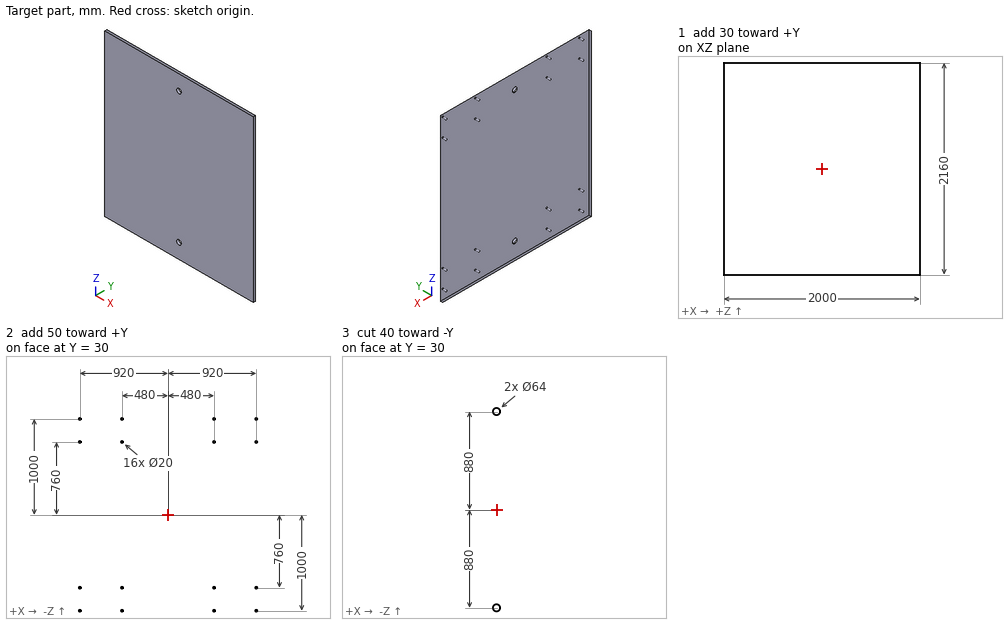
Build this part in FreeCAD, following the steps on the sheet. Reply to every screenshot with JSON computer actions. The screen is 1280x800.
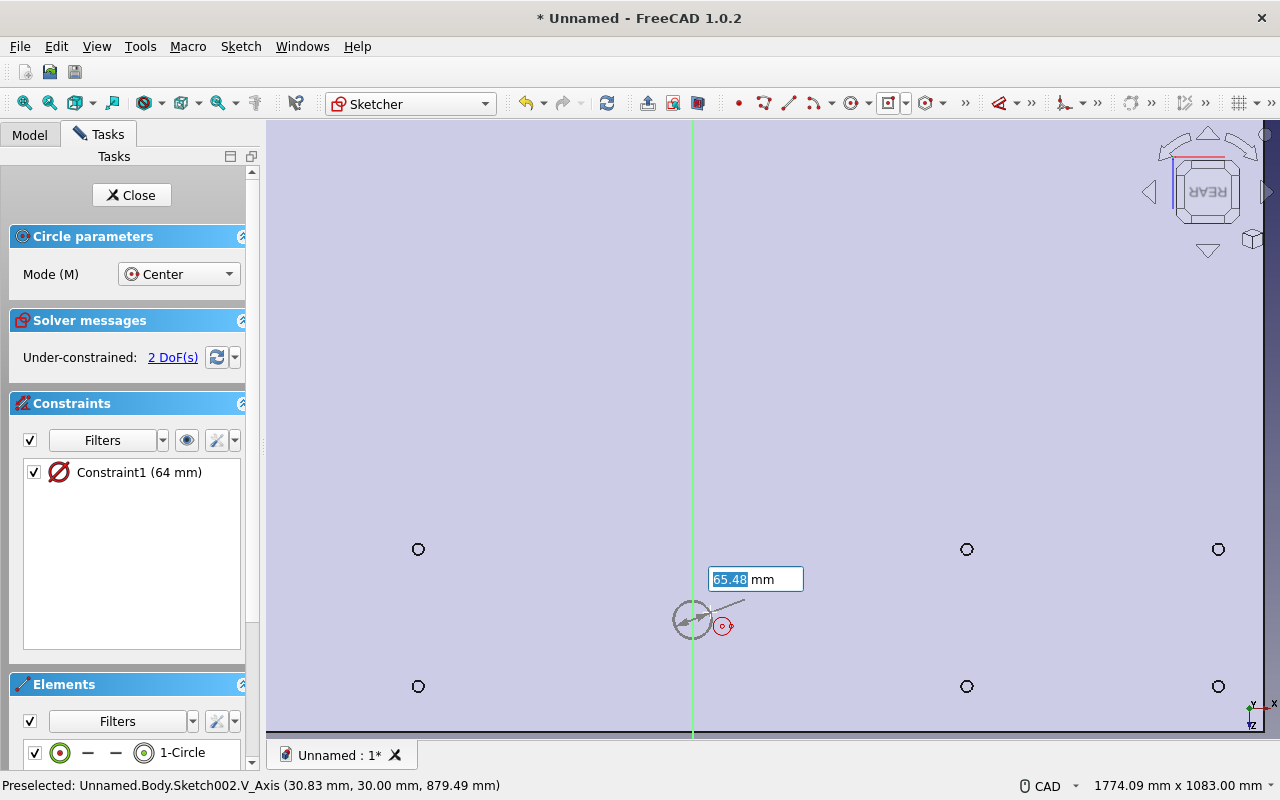
{"action": "type", "text": "64"}
{"action": "key", "text": "Return"}
{"action": "key", "text": "Escape"}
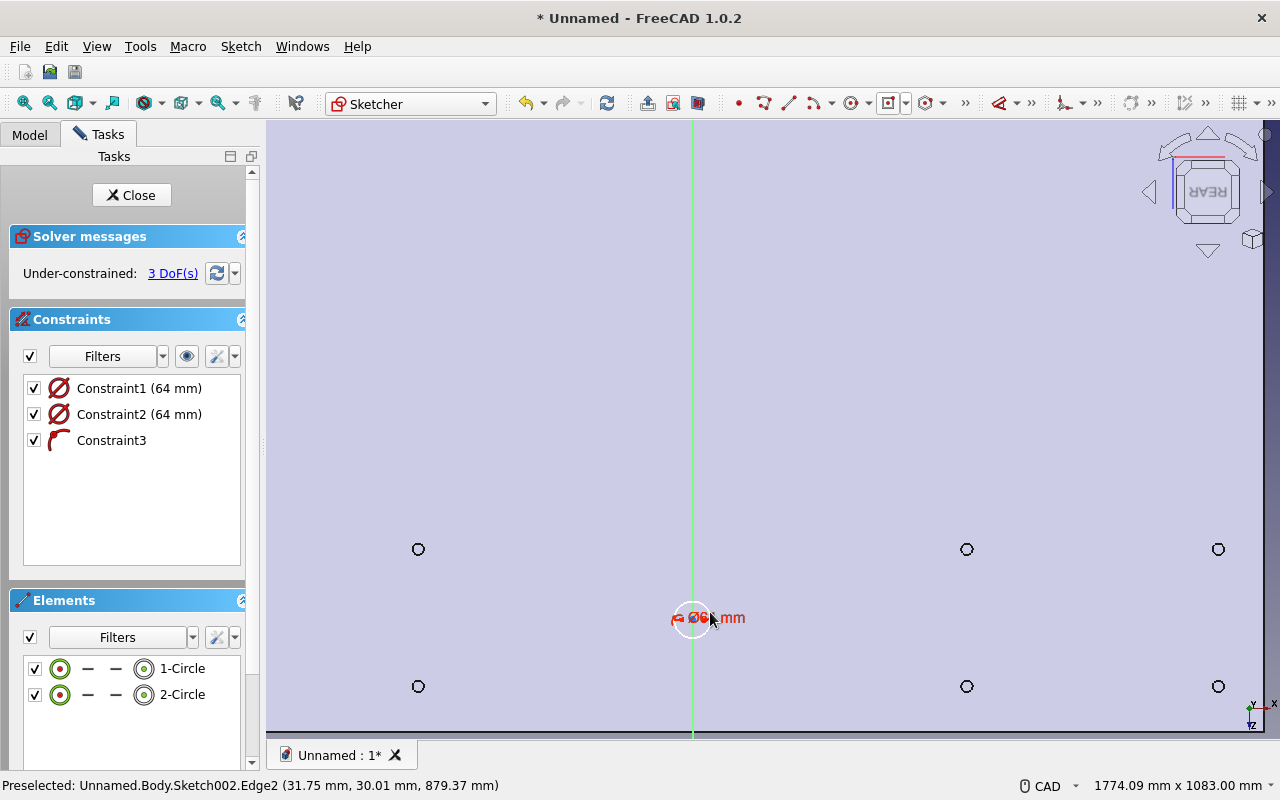
{"action": "scroll", "coordinate": [711, 613], "scroll_direction": "down", "scroll_amount": 5}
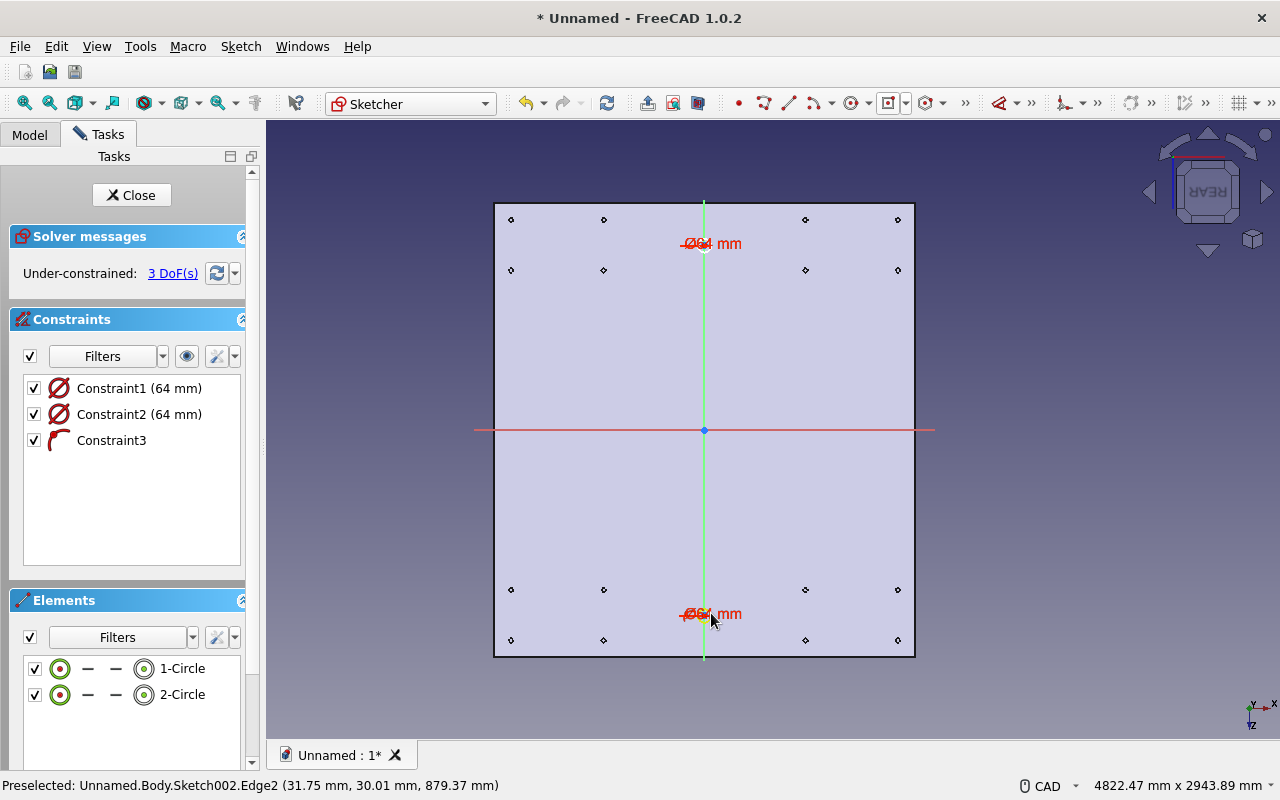
{"action": "left_click", "coordinate": [704, 246]}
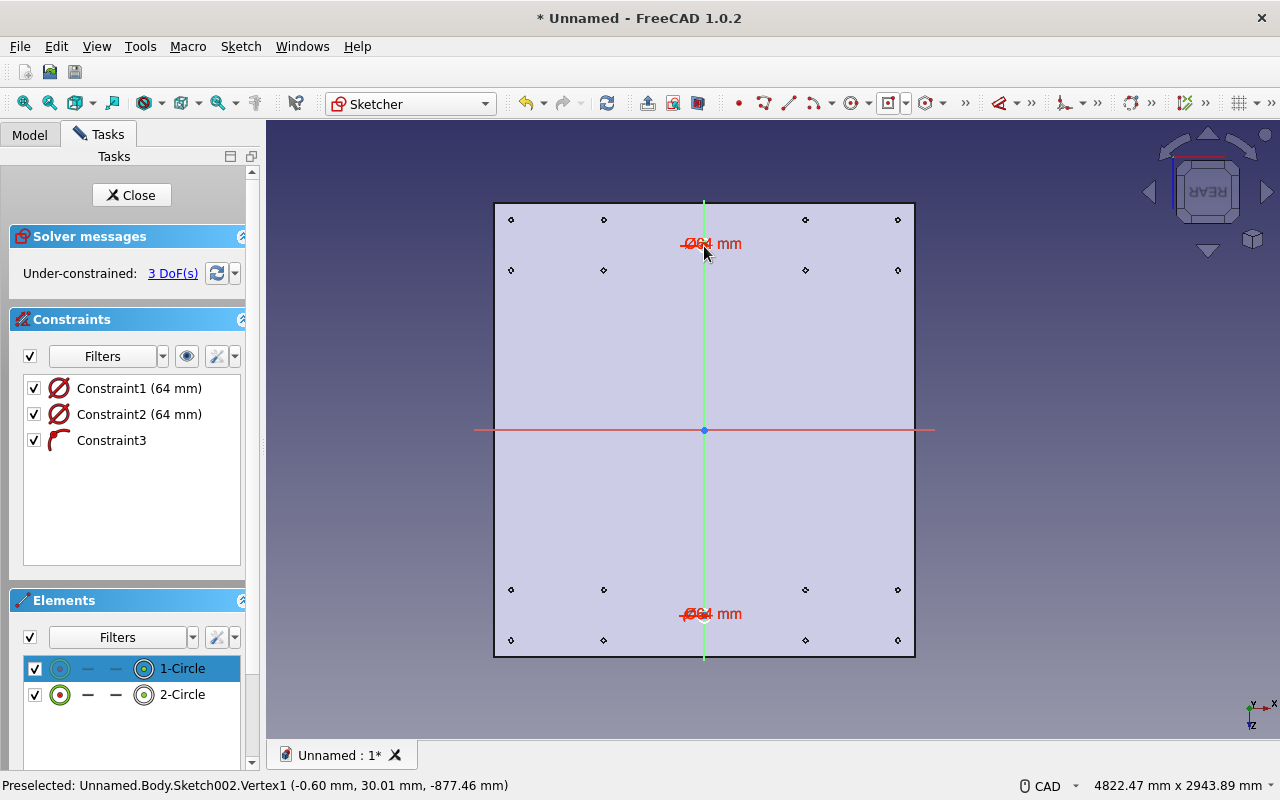
{"action": "left_click", "coordinate": [704, 550]}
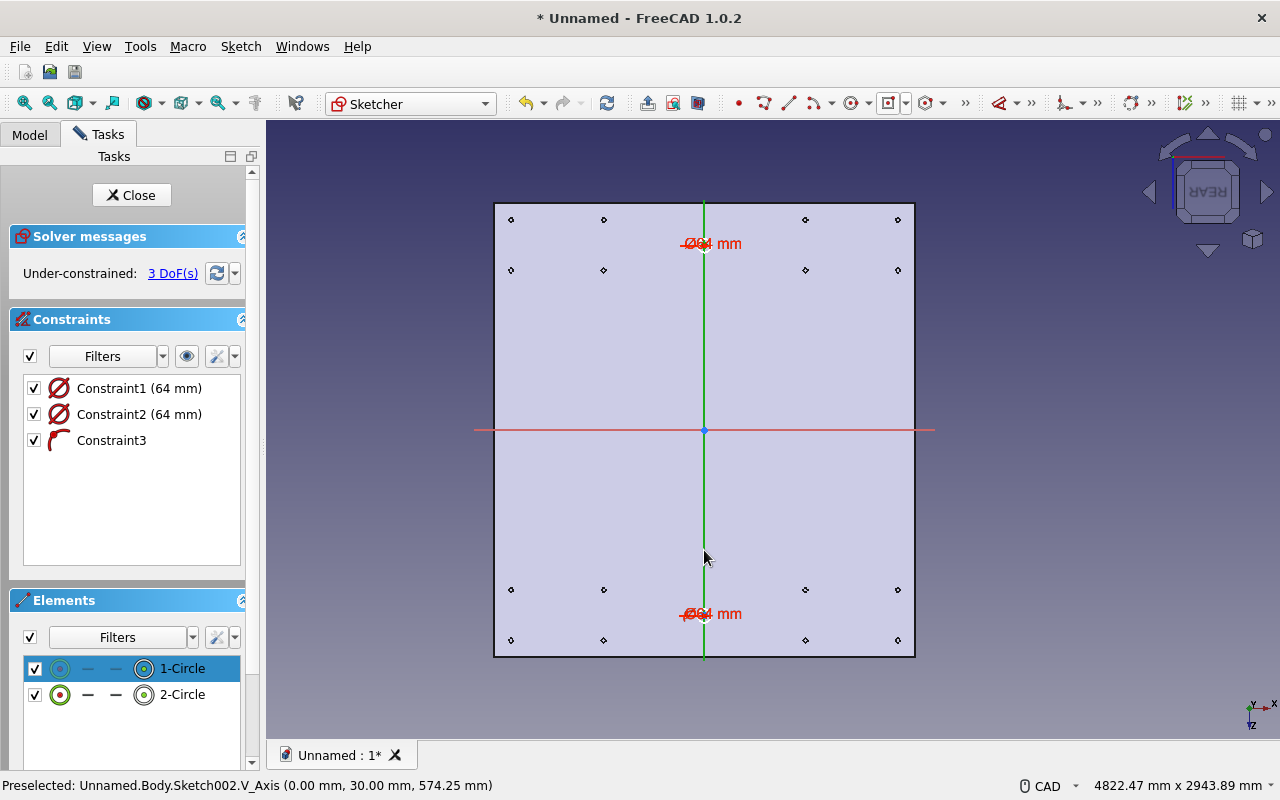
{"action": "key", "text": "c"}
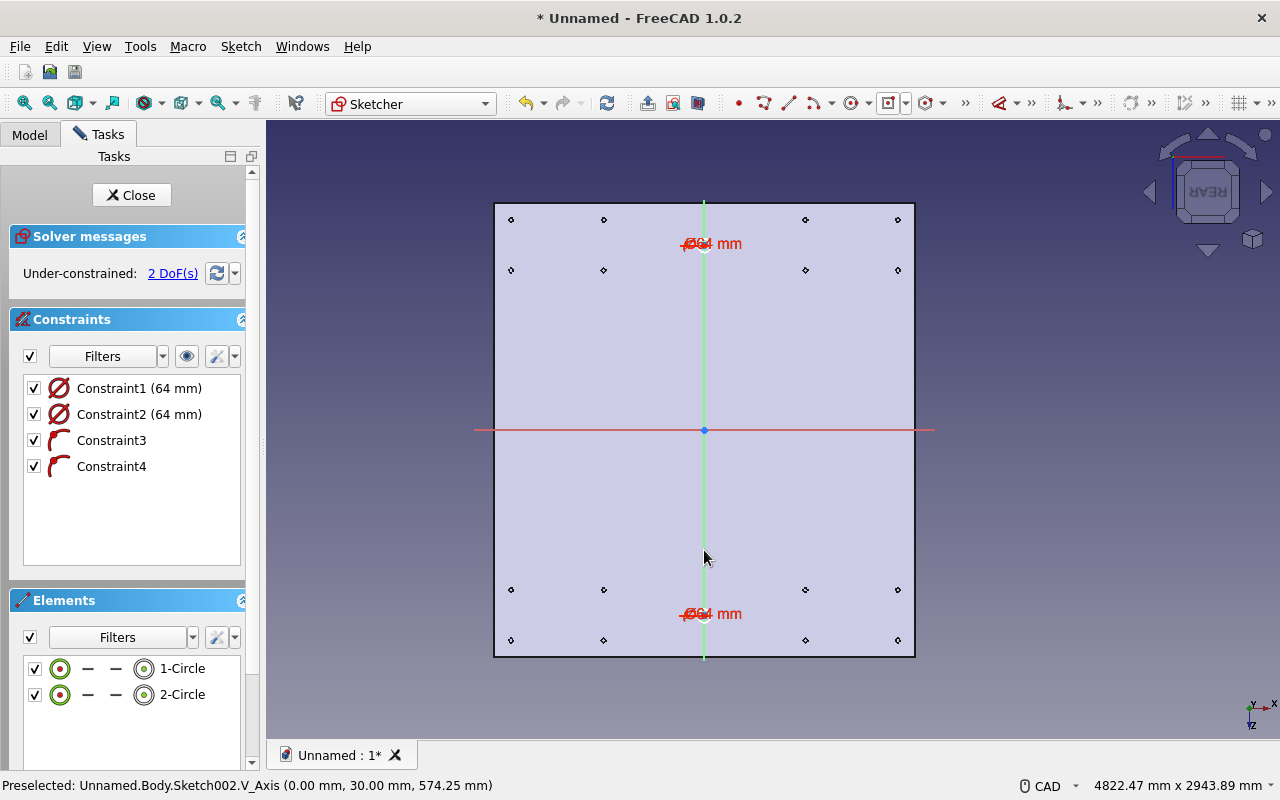
{"action": "left_click", "coordinate": [998, 104]}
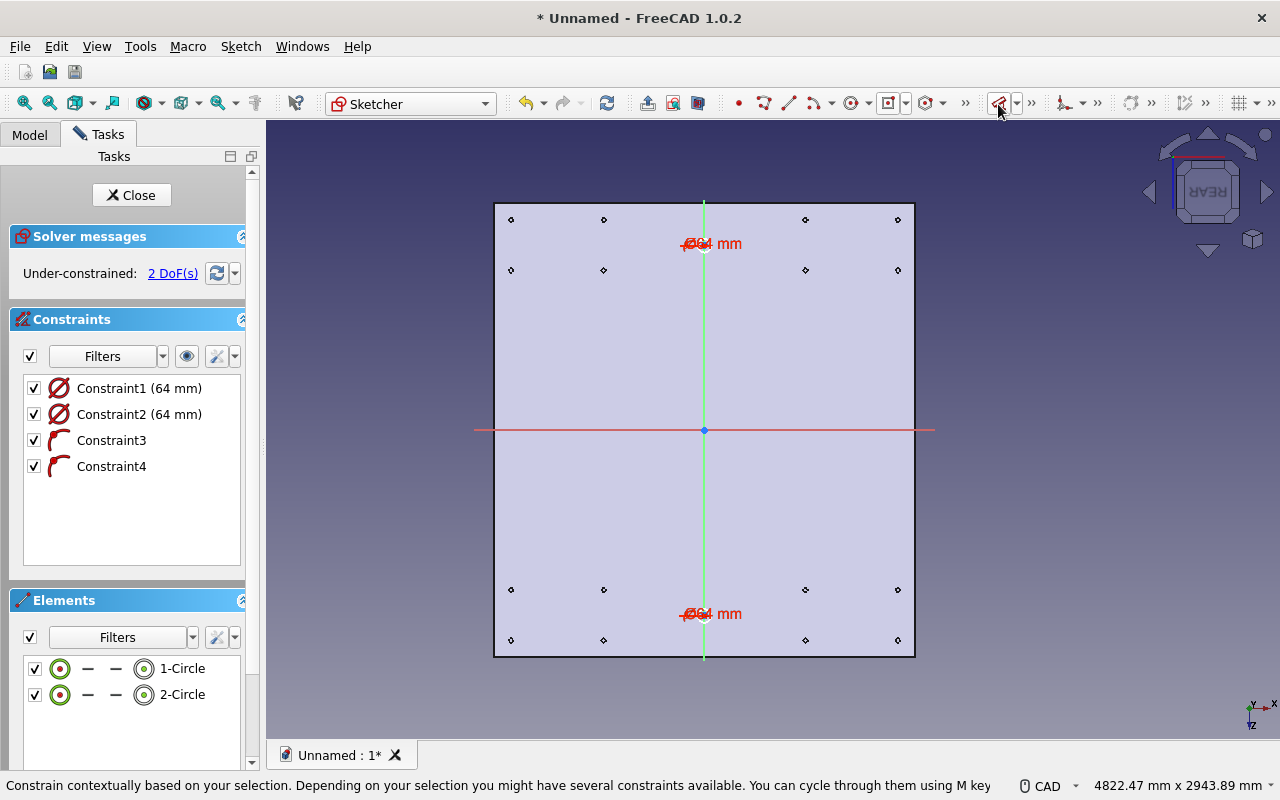
{"action": "left_click", "coordinate": [704, 246]}
{"action": "left_click", "coordinate": [738, 338]}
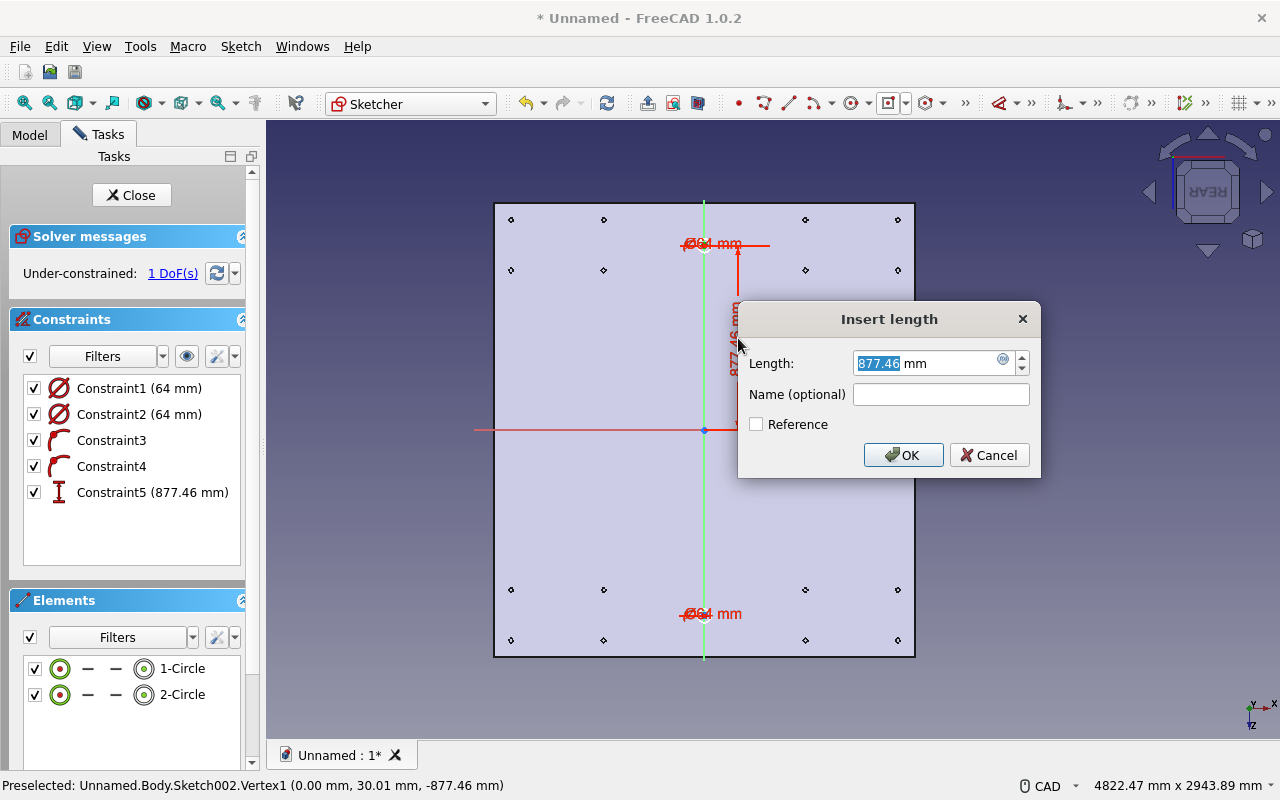
{"action": "type", "text": "880"}
{"action": "key", "text": "Return"}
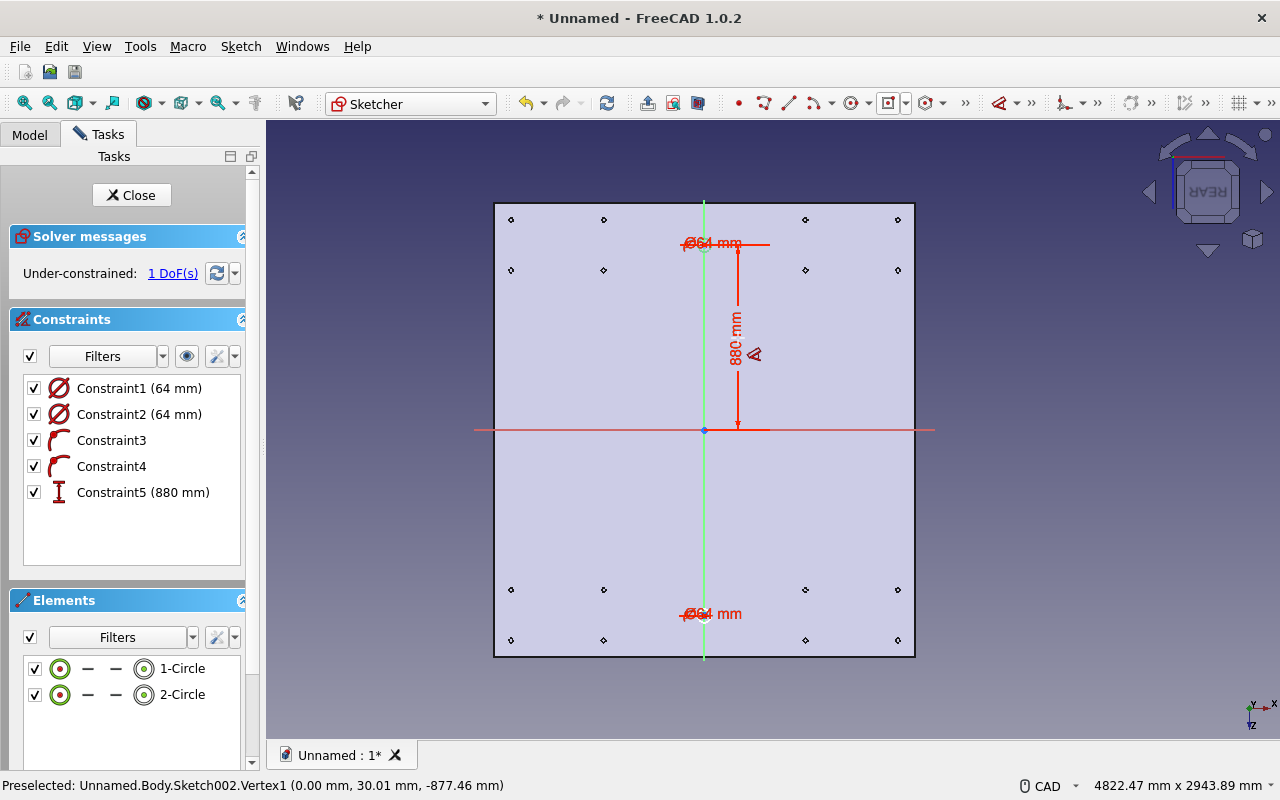
{"action": "left_click", "coordinate": [704, 616]}
{"action": "left_click", "coordinate": [738, 523]}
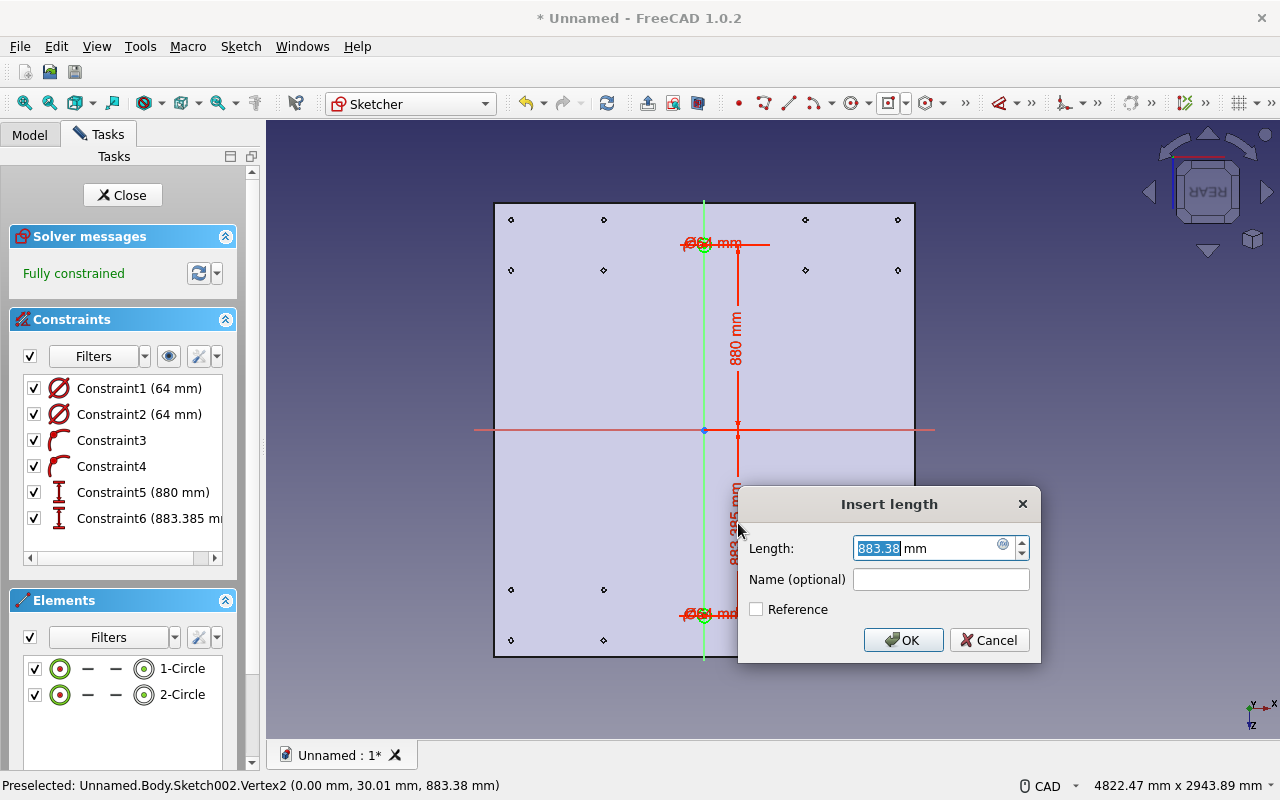
{"action": "type", "text": "880"}
{"action": "key", "text": "Return"}
{"action": "key", "text": "Escape"}